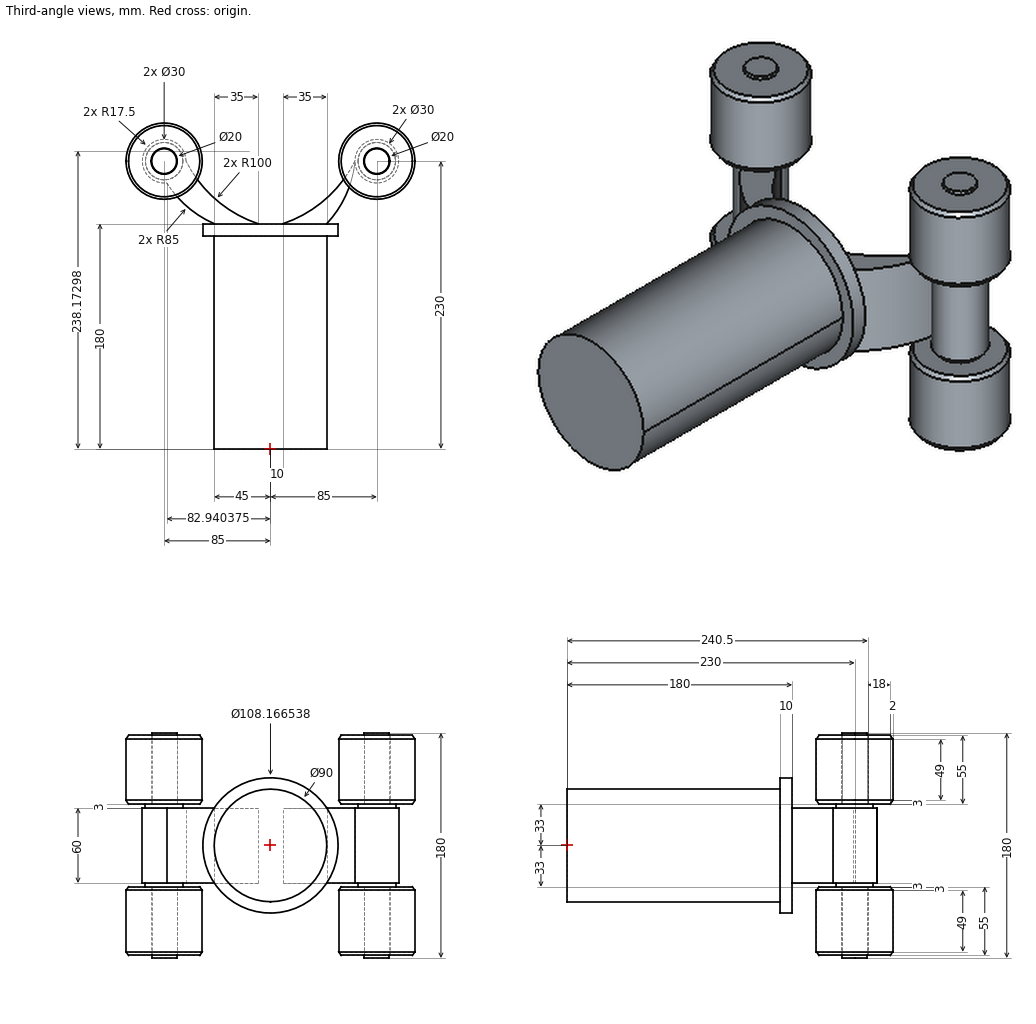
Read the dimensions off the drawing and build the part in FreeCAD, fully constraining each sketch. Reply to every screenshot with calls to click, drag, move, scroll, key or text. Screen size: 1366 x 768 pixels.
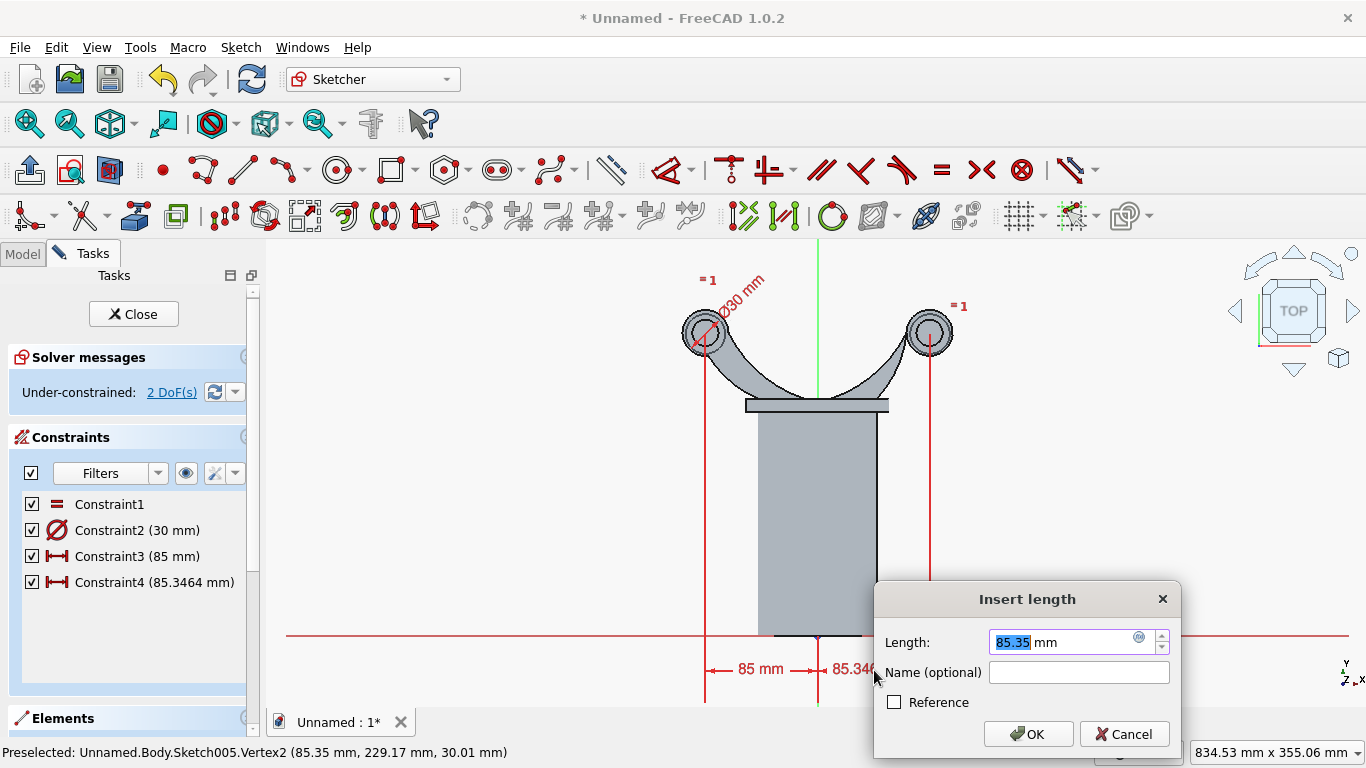
text(85)
key(Return)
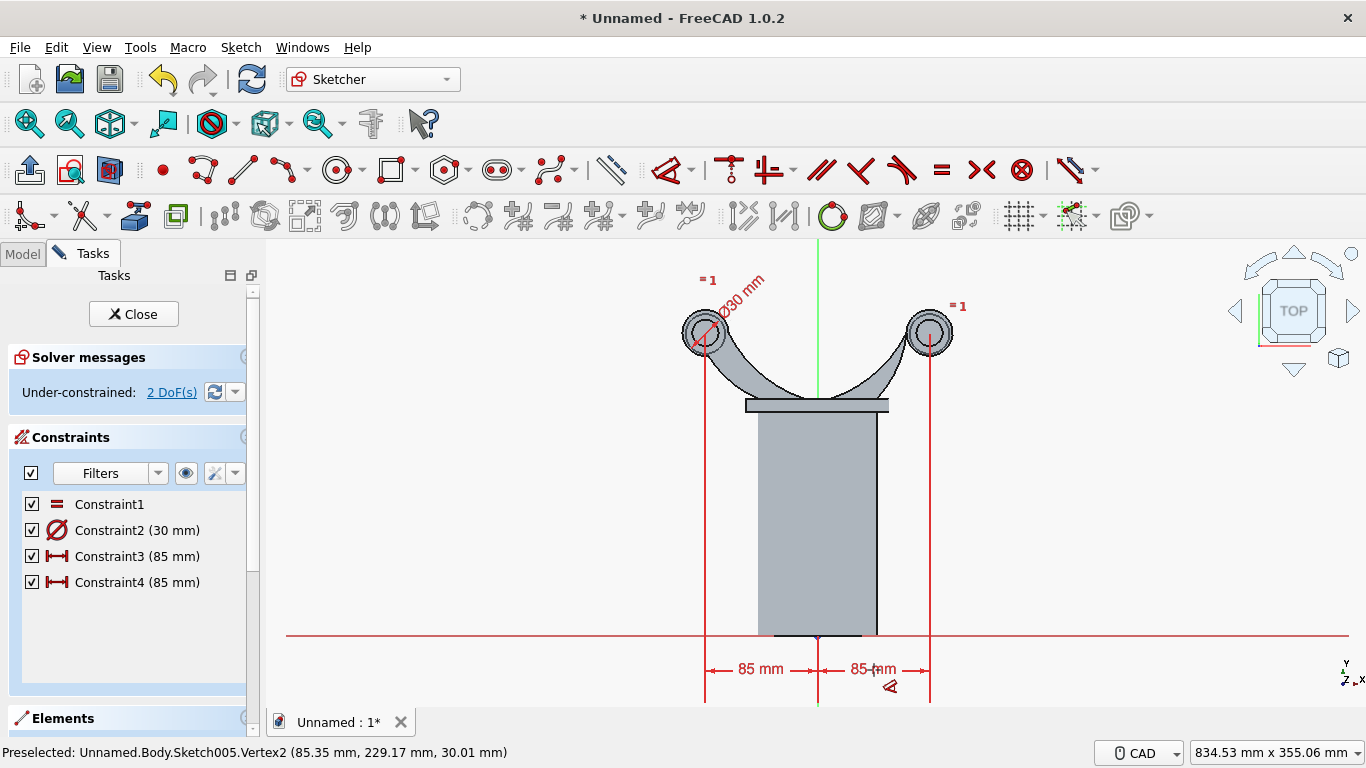
click(705, 334)
click(671, 485)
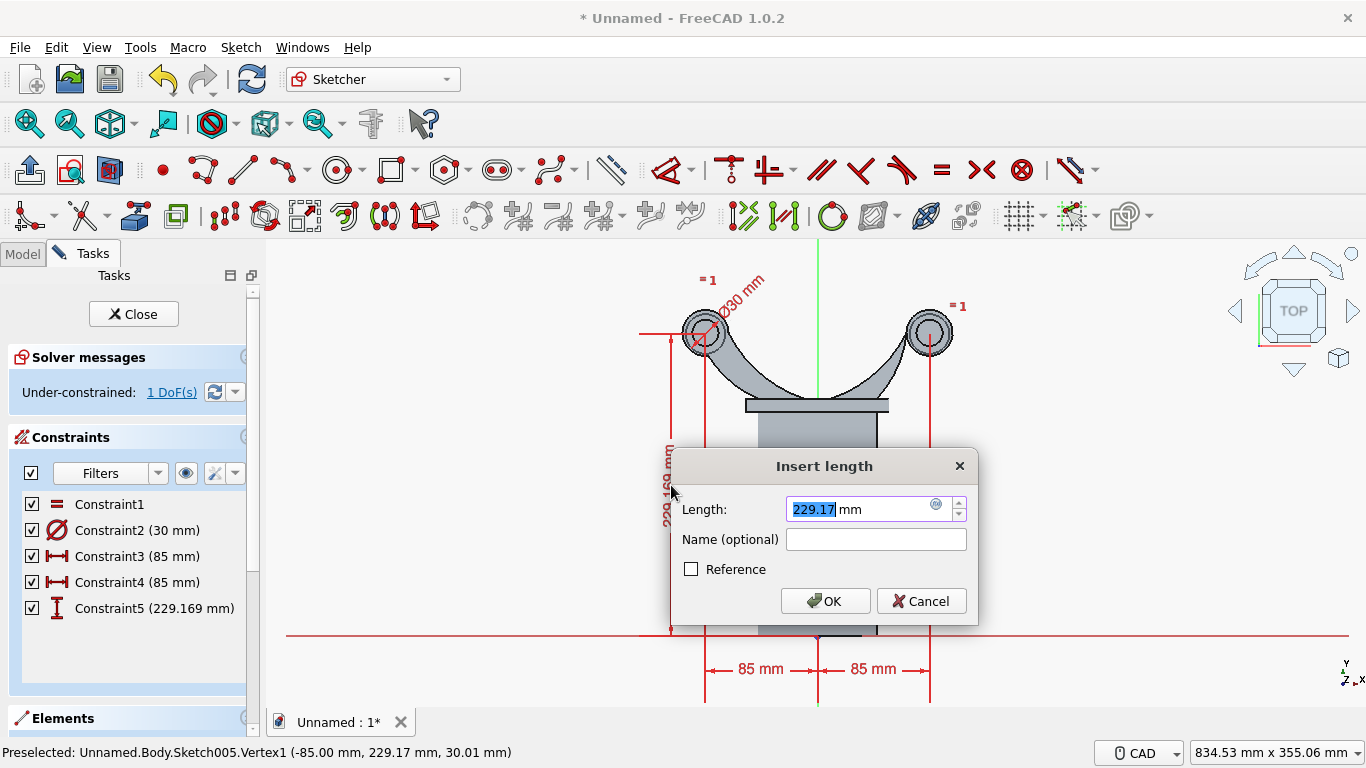
text(230)
key(Return)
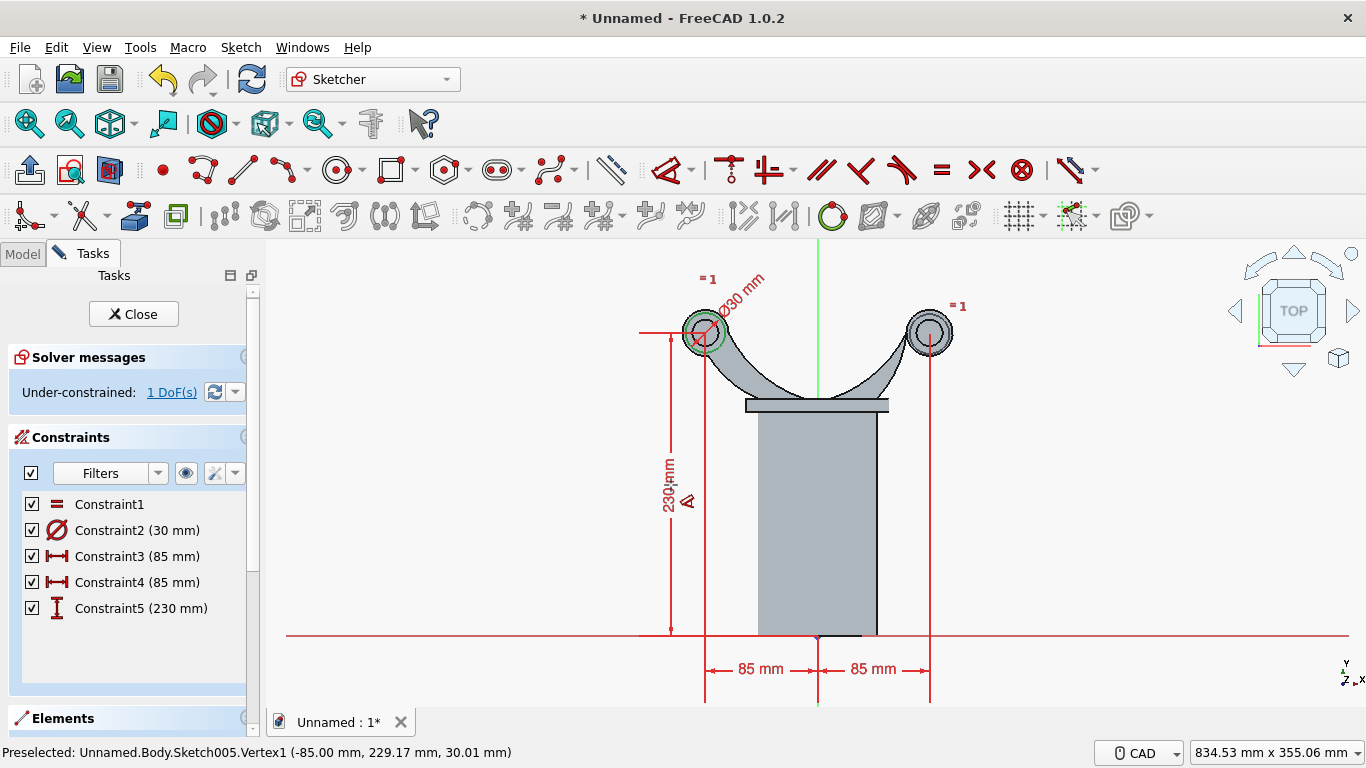
click(930, 334)
click(964, 485)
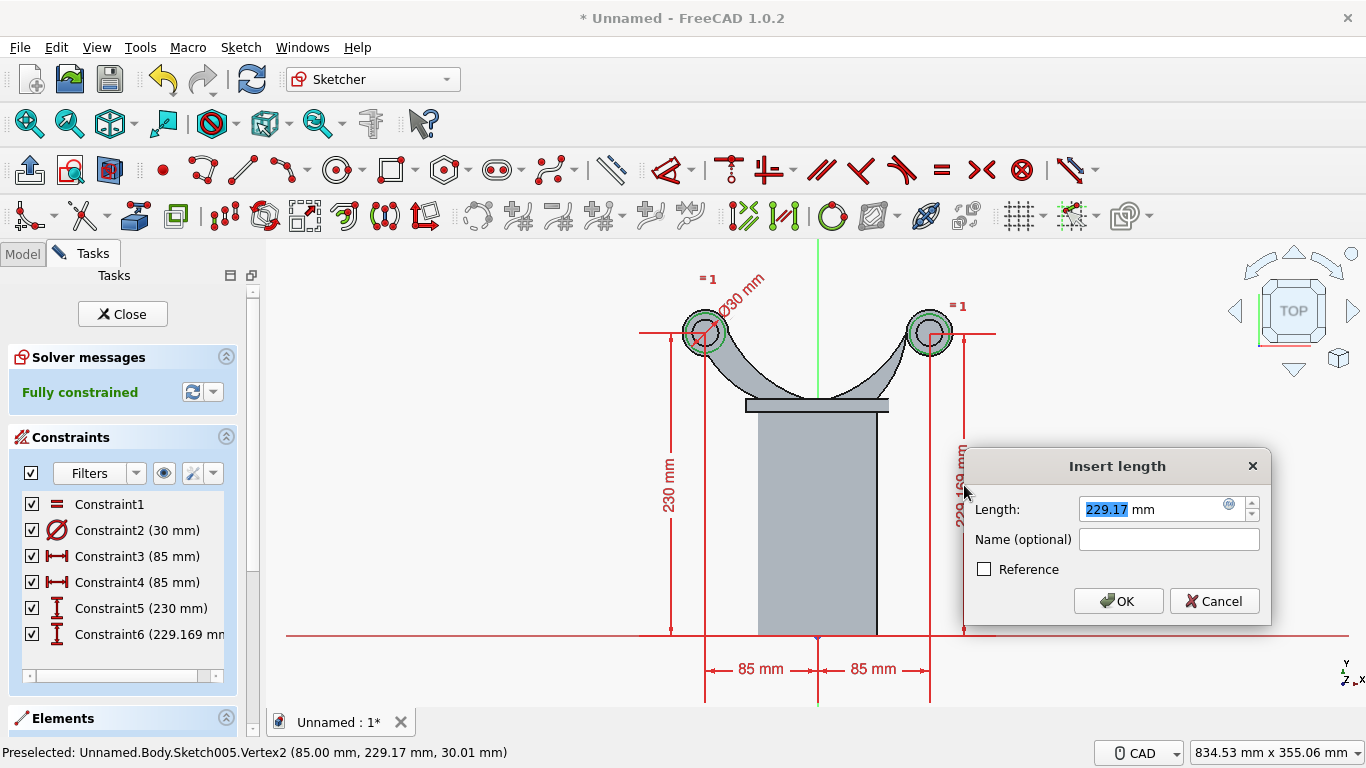
text(230)
key(Return)
key(Escape)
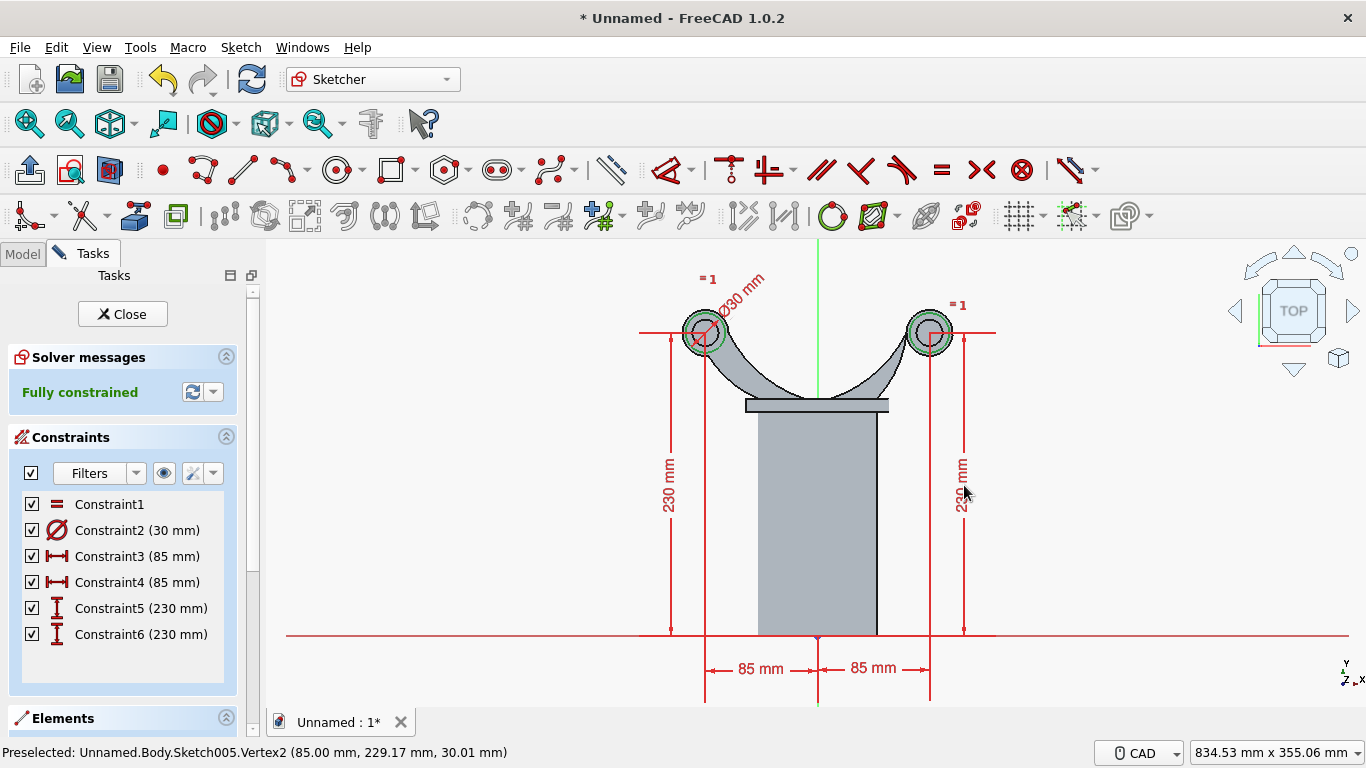
click(123, 314)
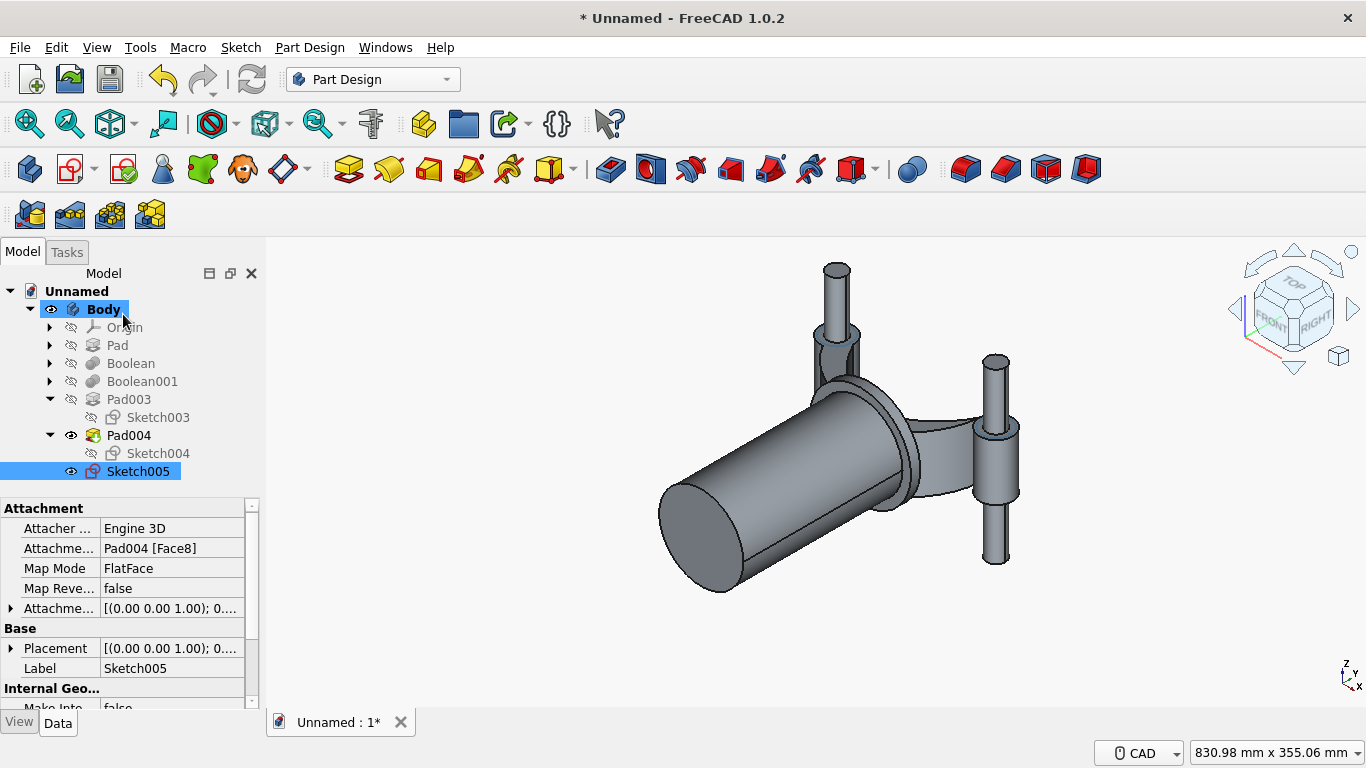
click(350, 170)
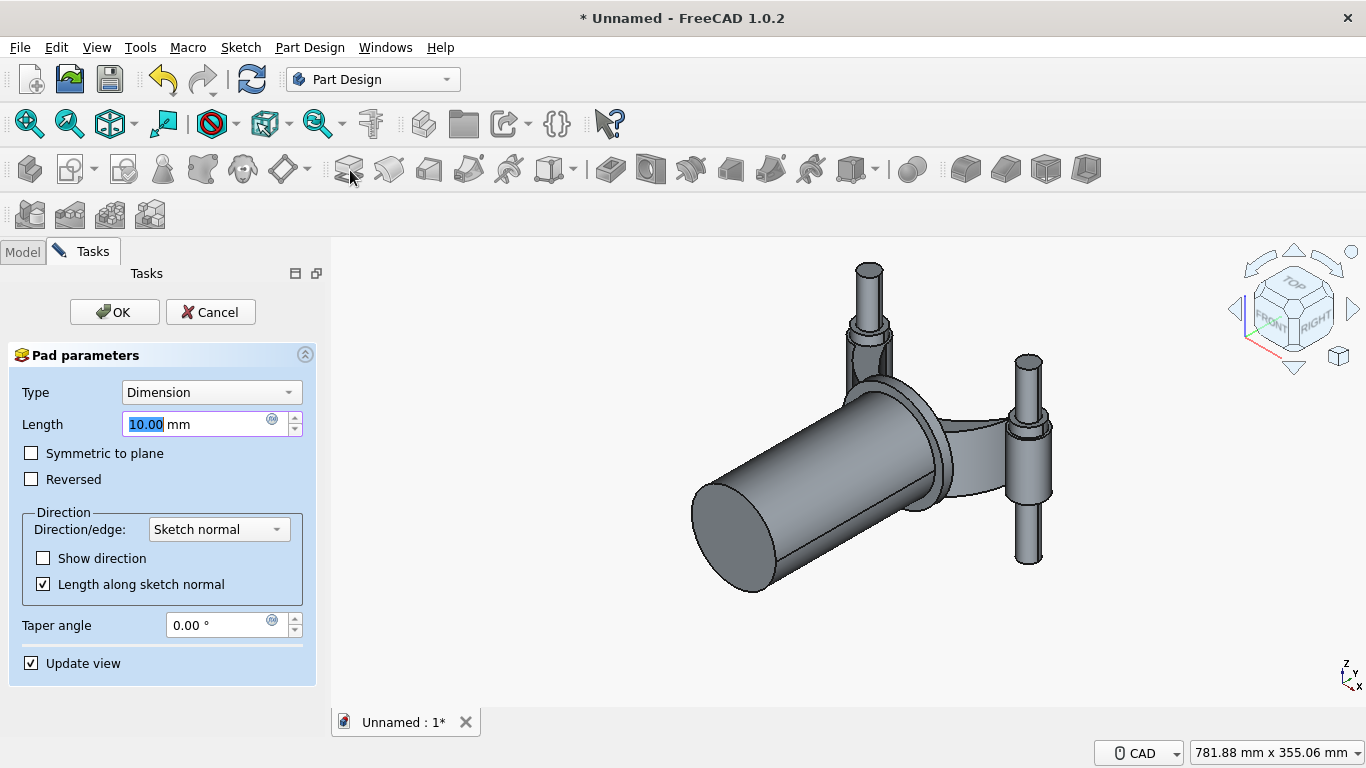
text(3)
key(Tab)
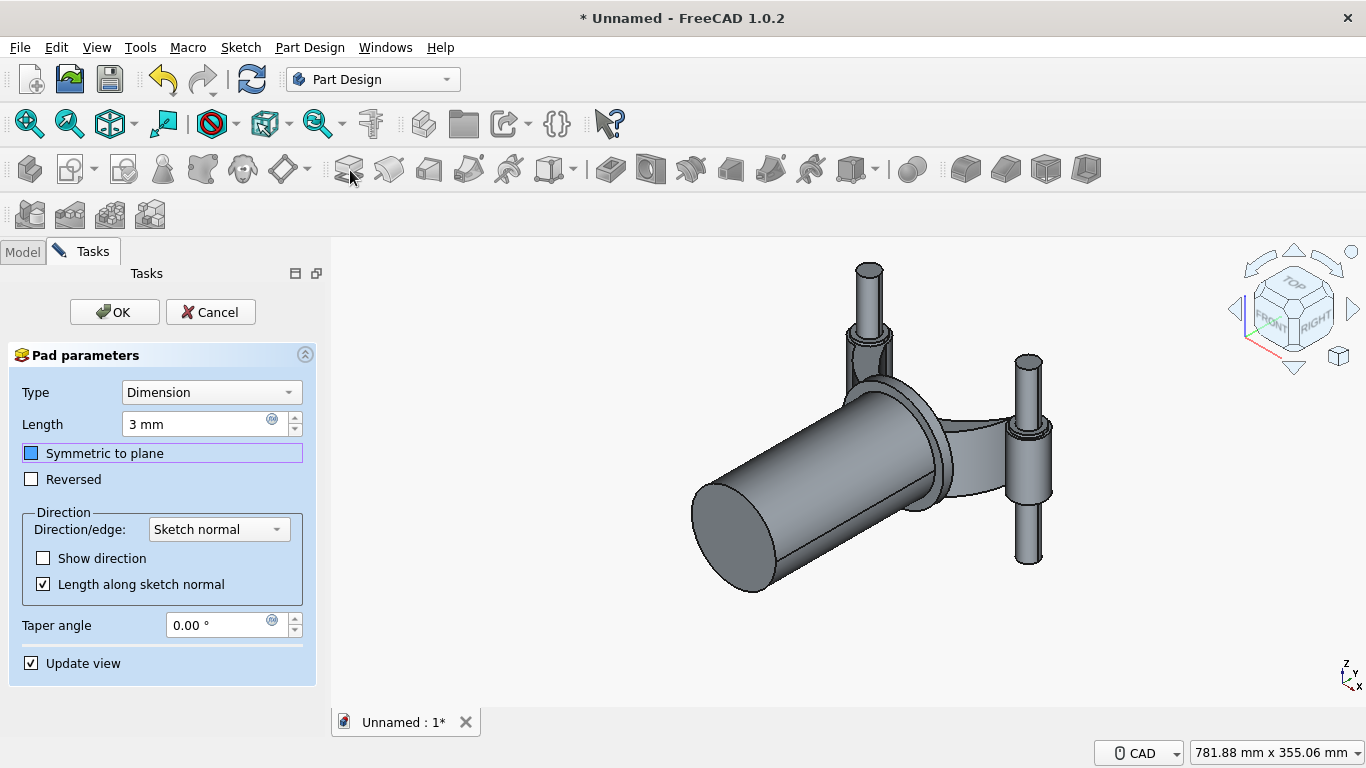
click(115, 312)